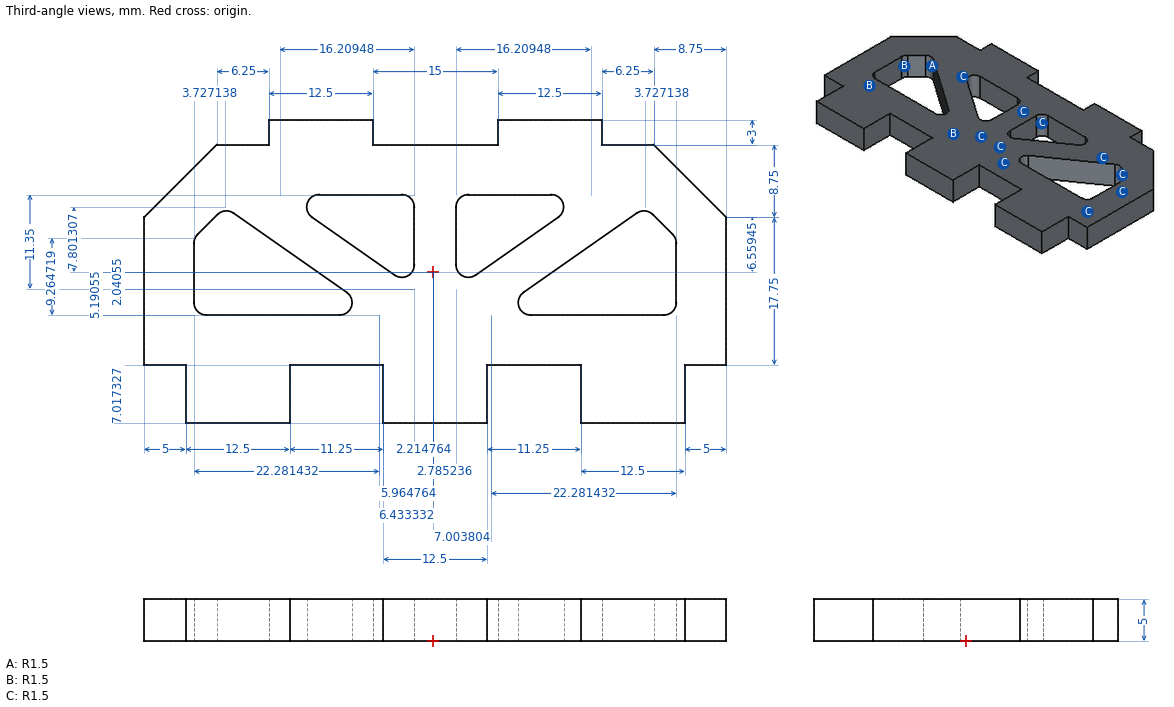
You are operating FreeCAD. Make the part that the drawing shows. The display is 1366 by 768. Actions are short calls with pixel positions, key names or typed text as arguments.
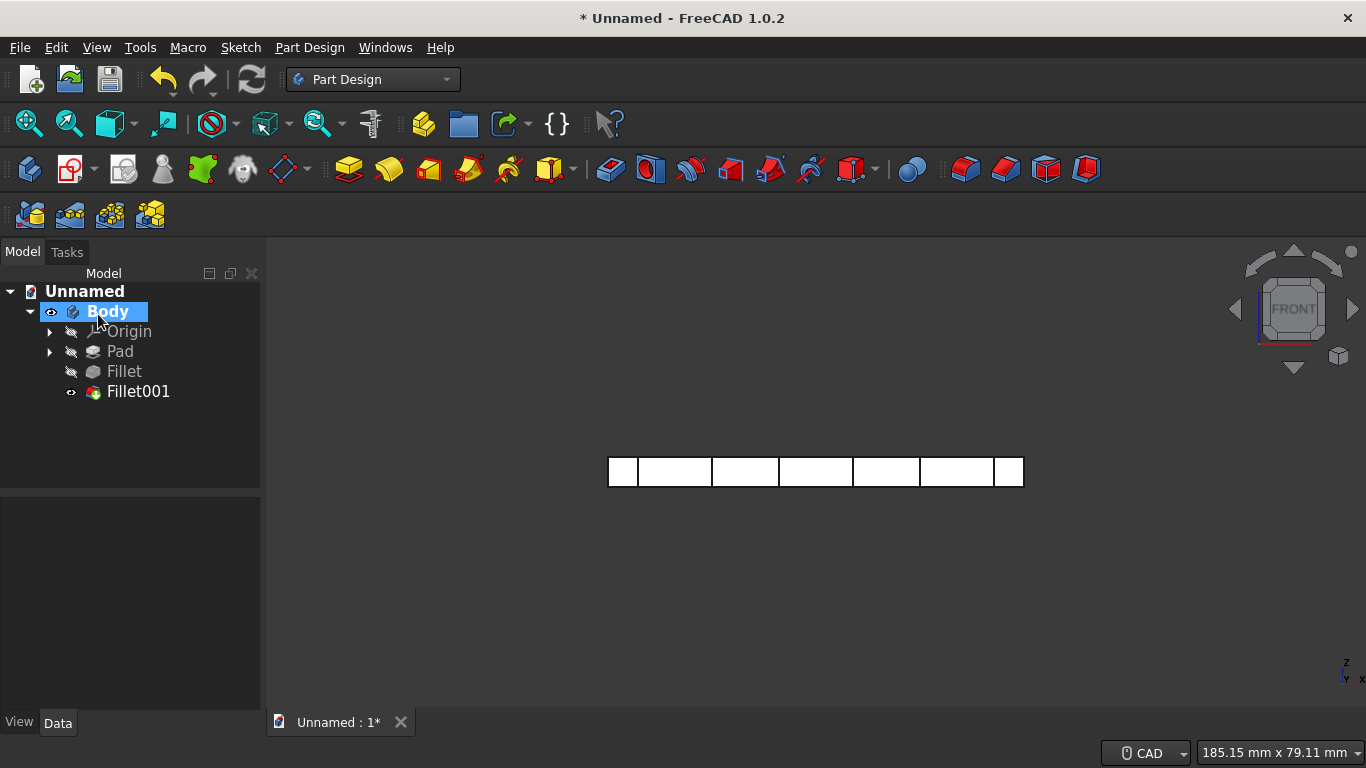
key(3)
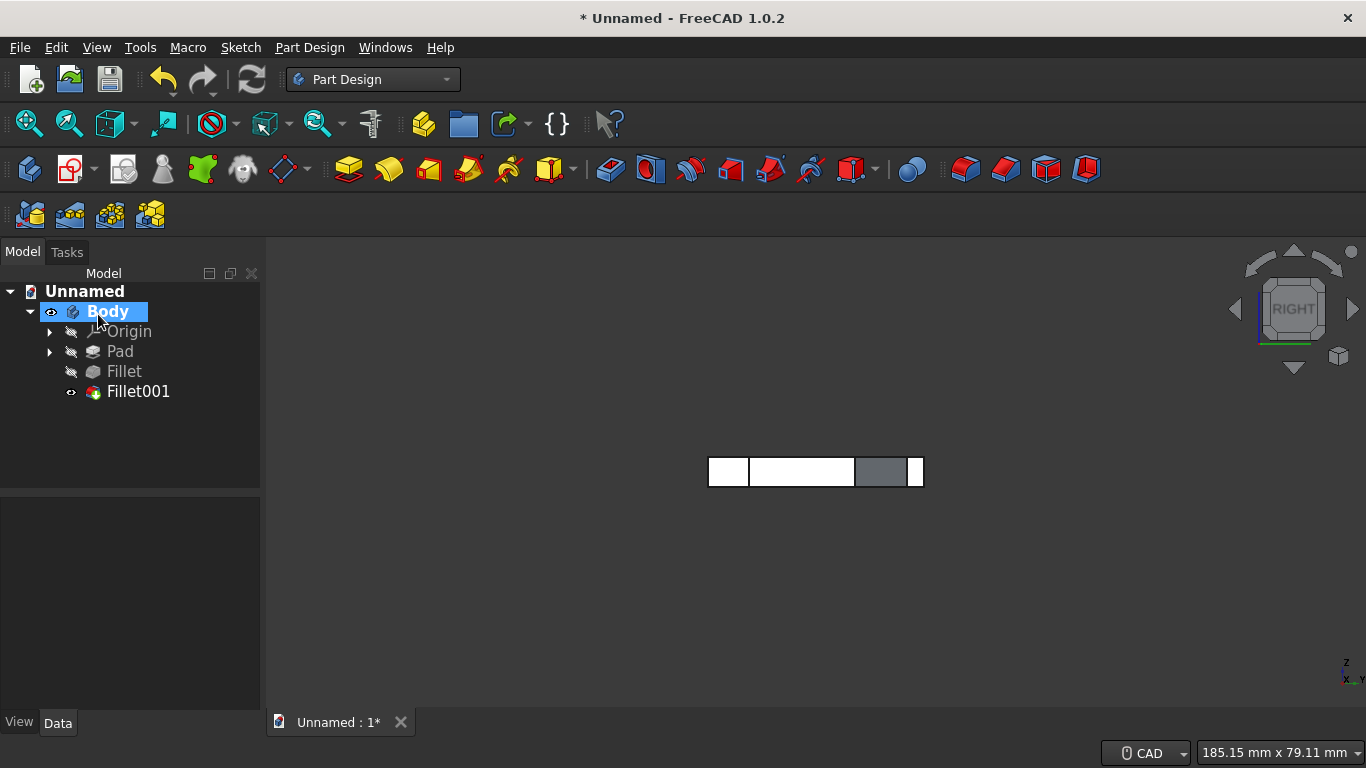
click(30, 124)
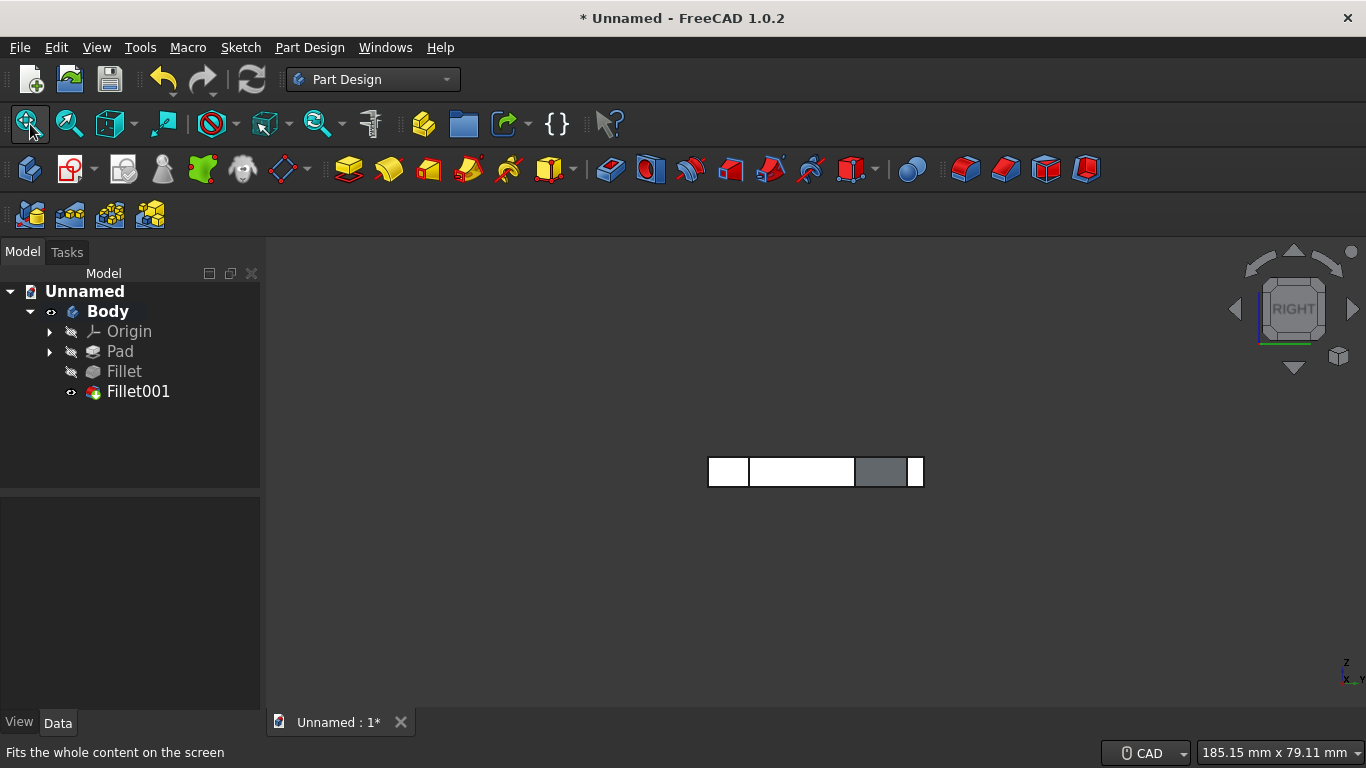
key(5)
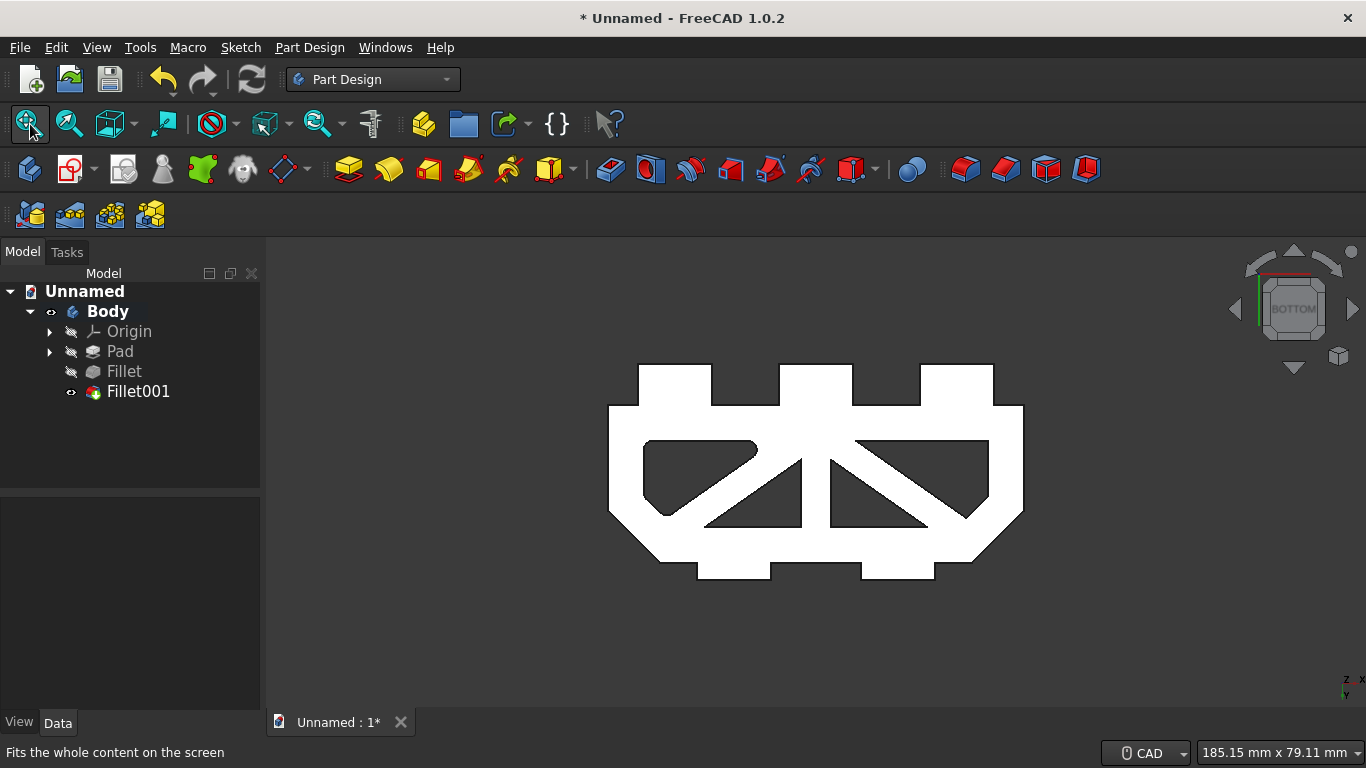
key(4)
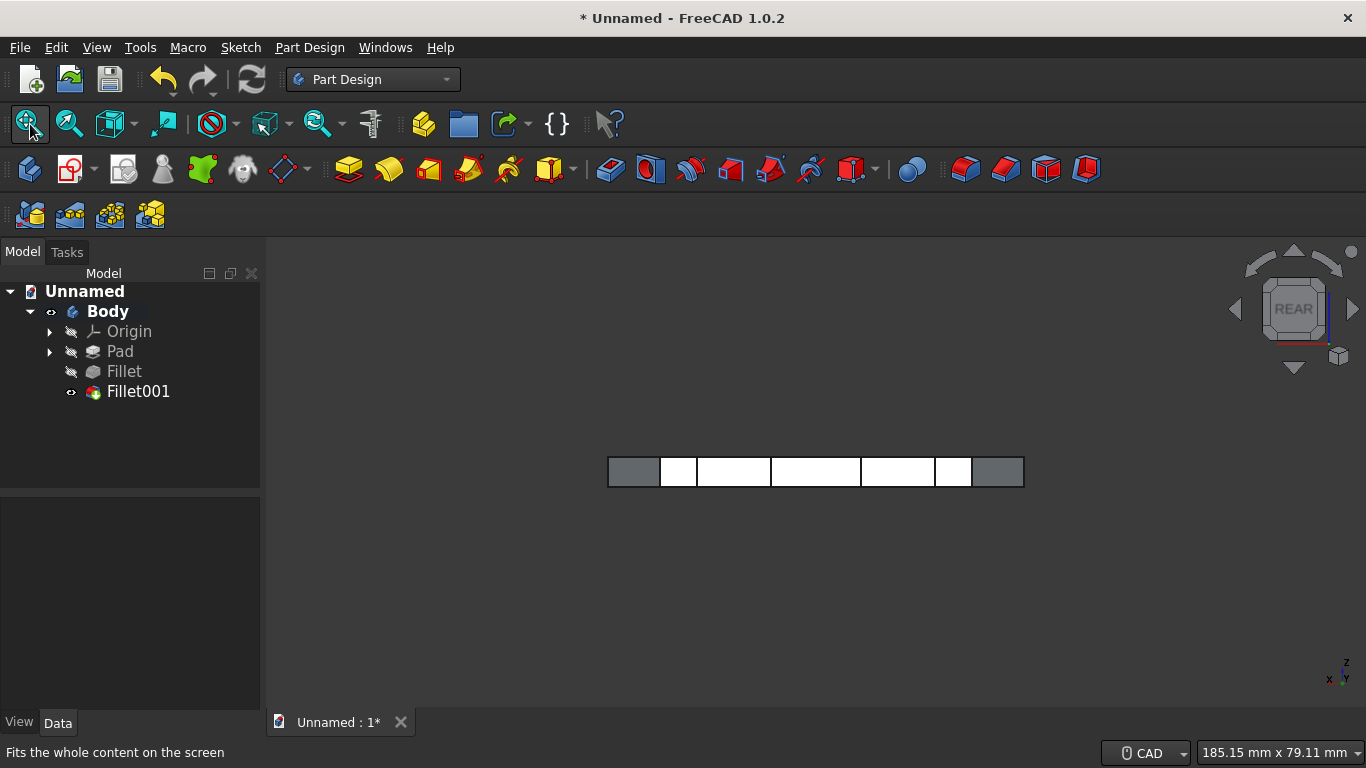
key(v)
key(f)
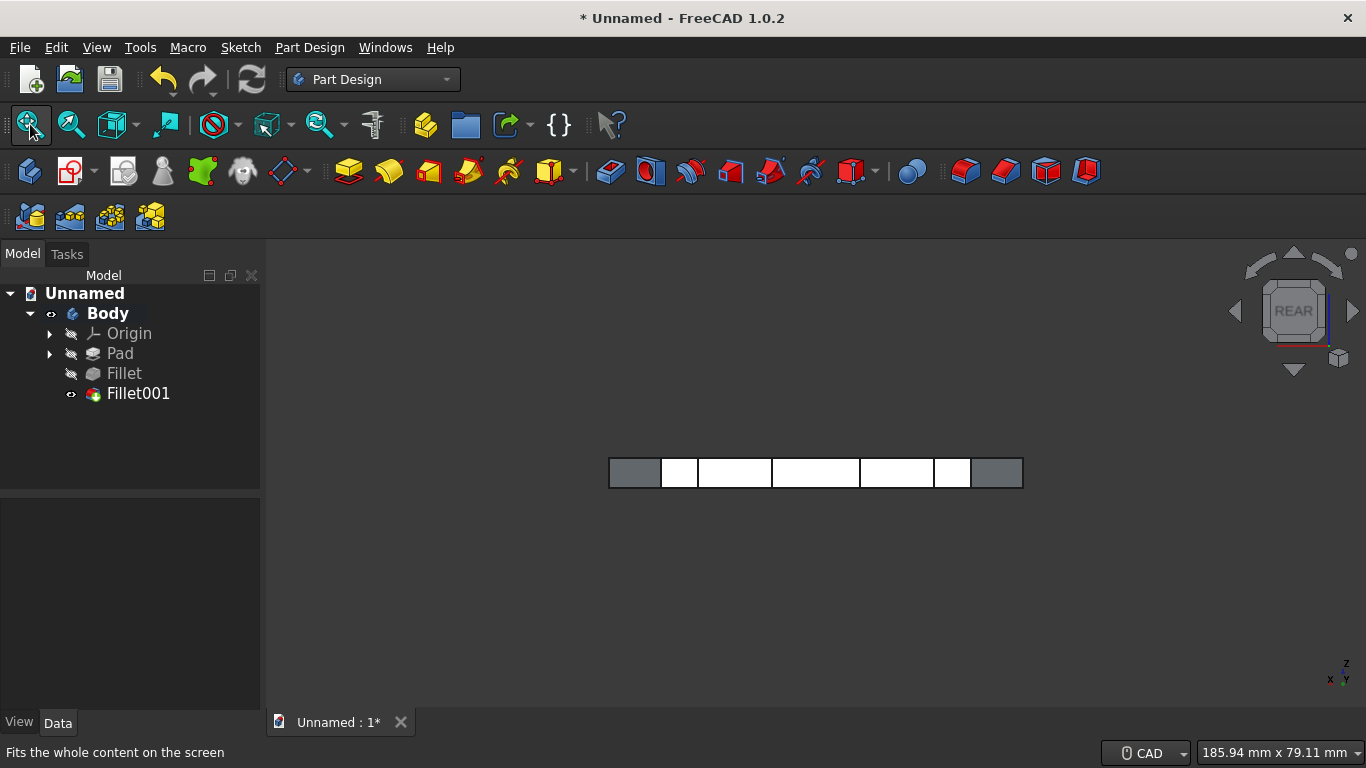
key(6)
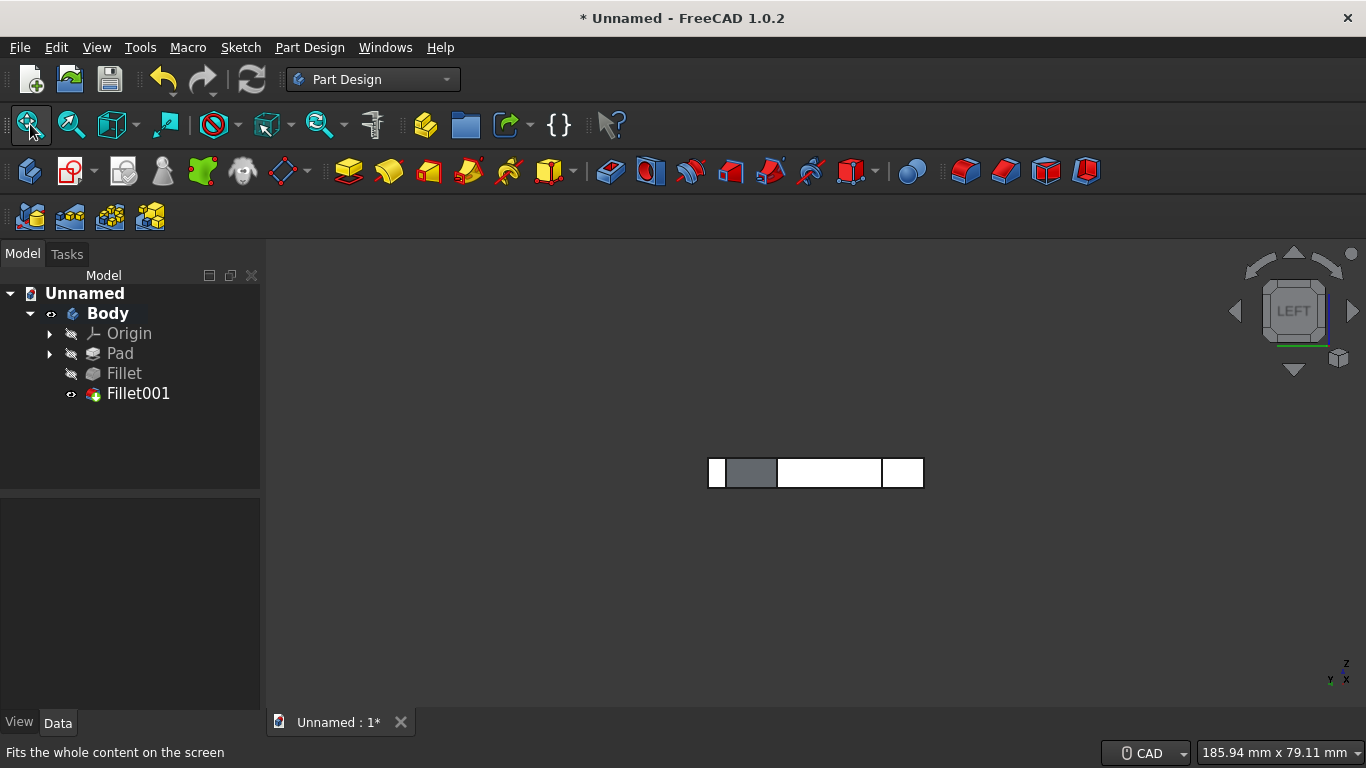
key(v)
key(f)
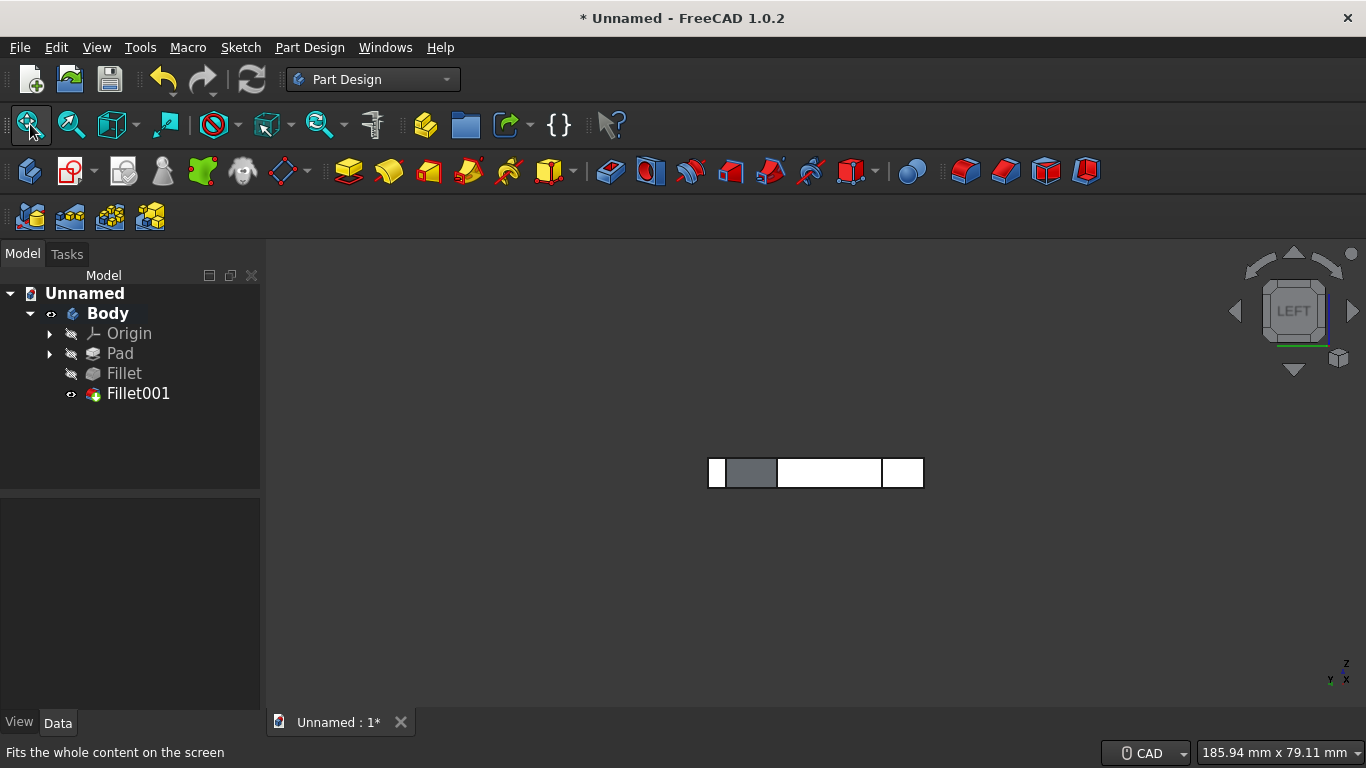
key(v)
key(3)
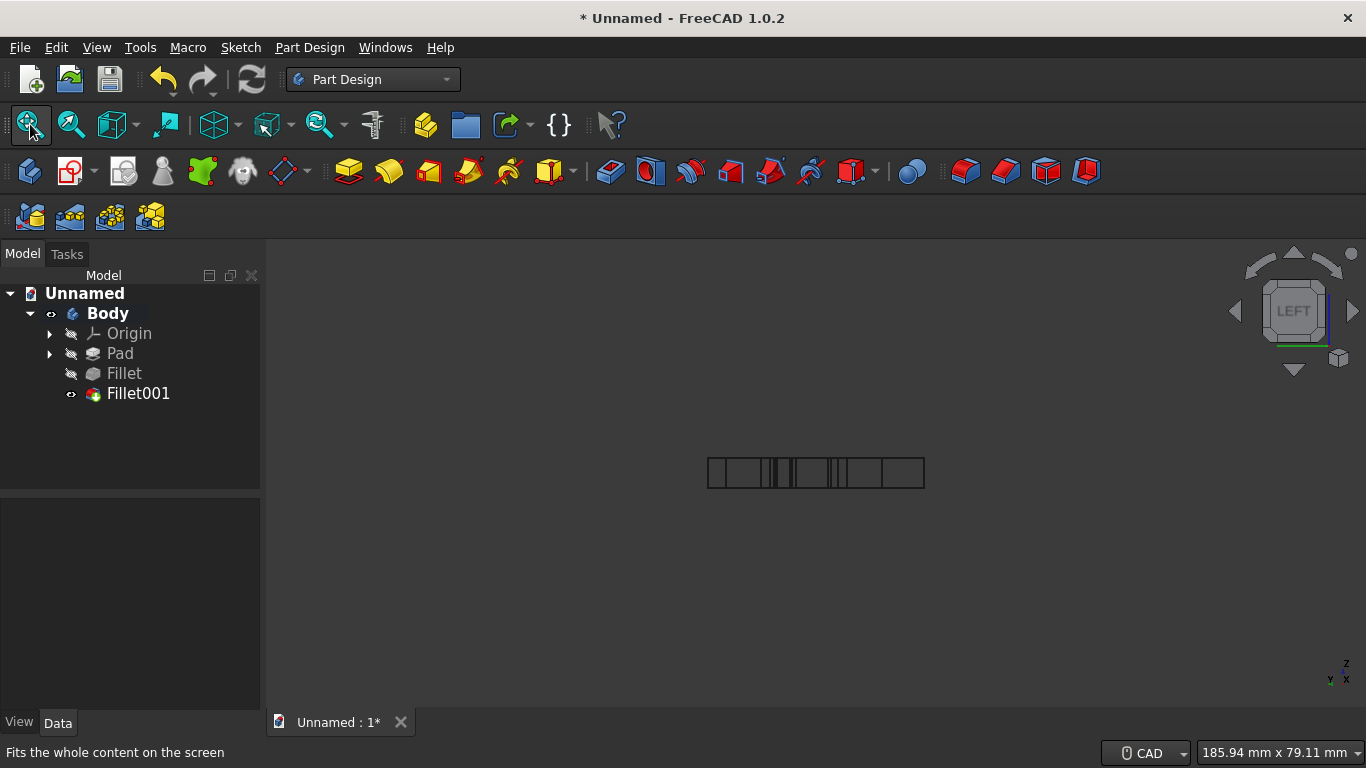
key(0)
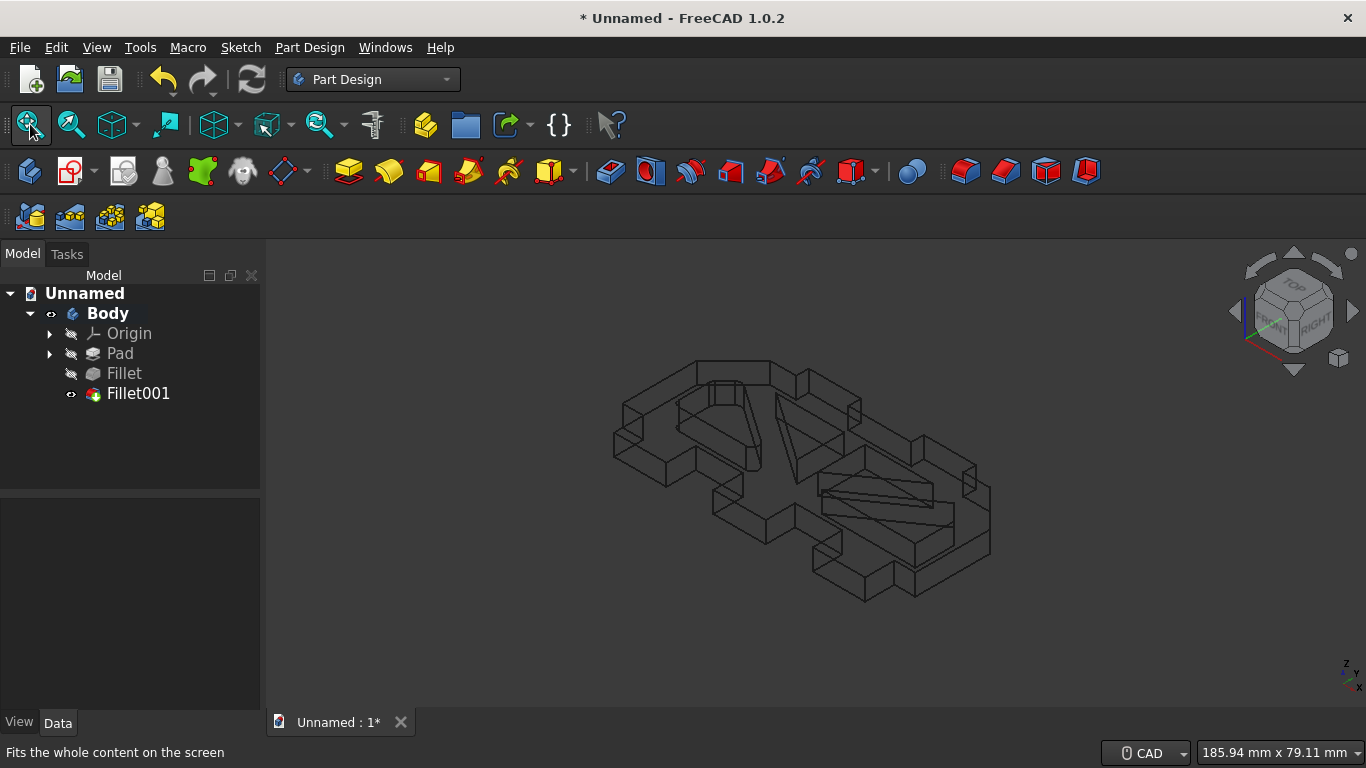
click(915, 555)